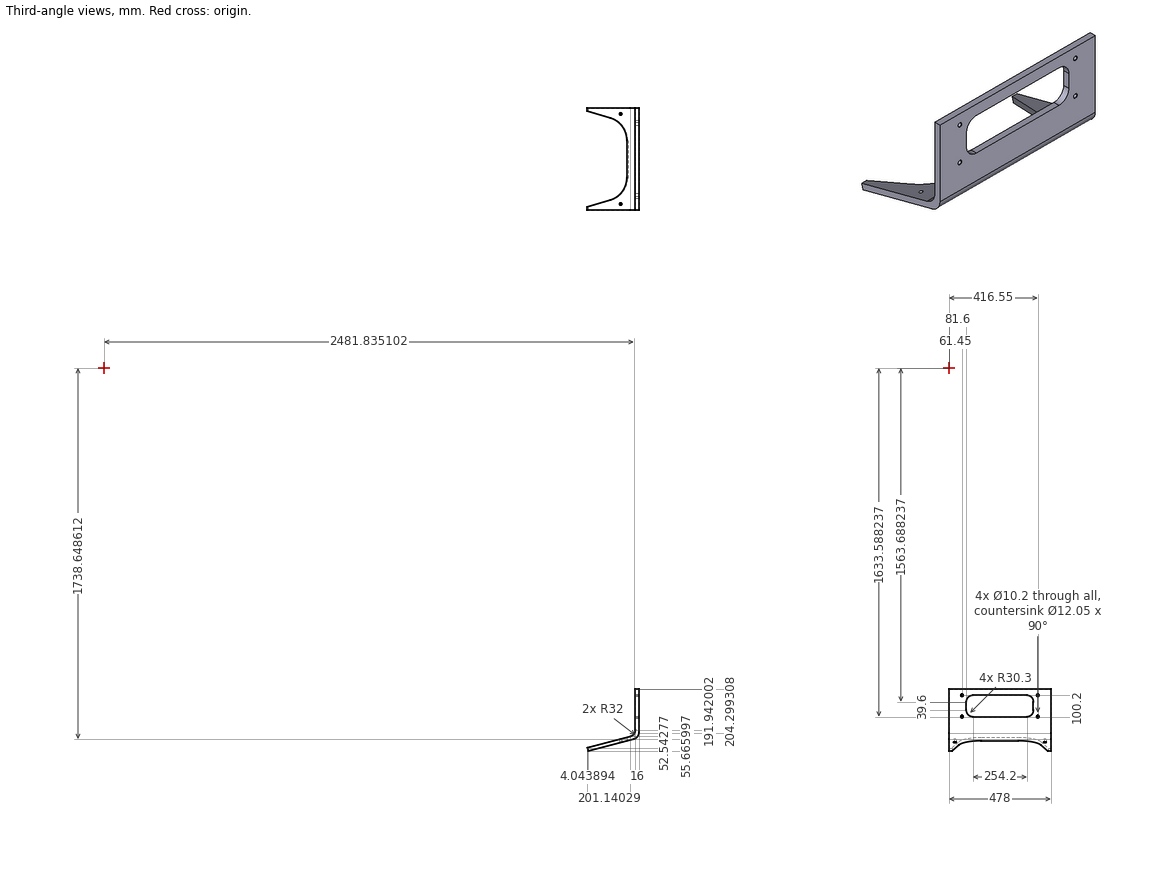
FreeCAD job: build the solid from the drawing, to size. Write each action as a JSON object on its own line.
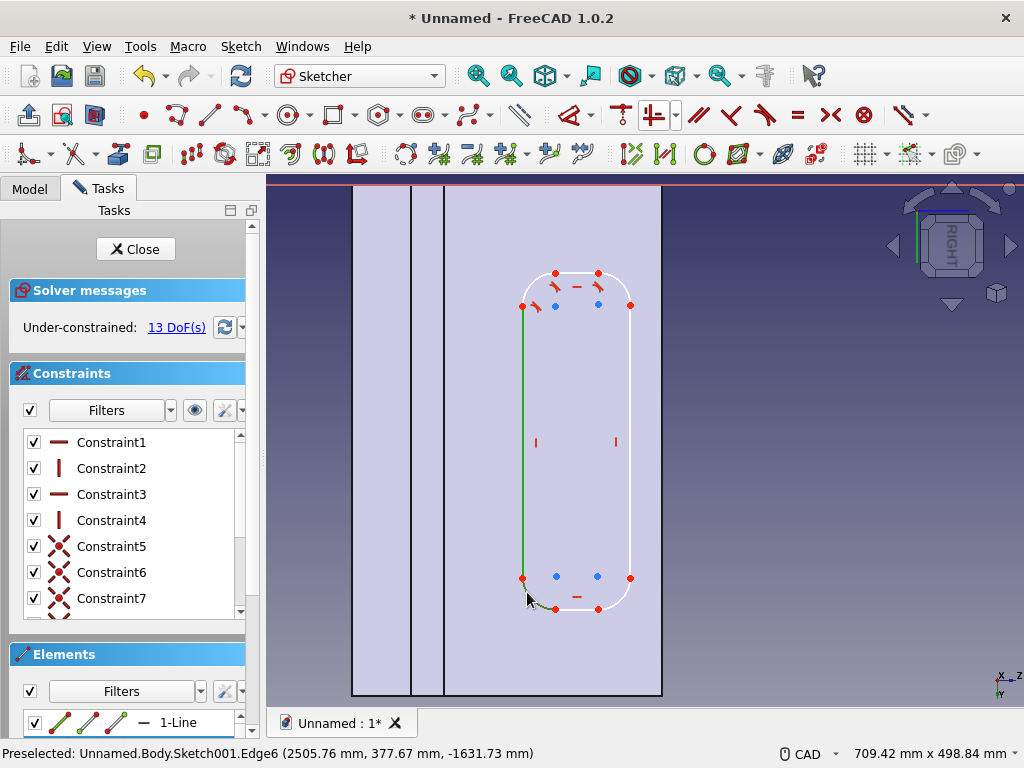
{"action": "left_click", "coordinate": [765, 116]}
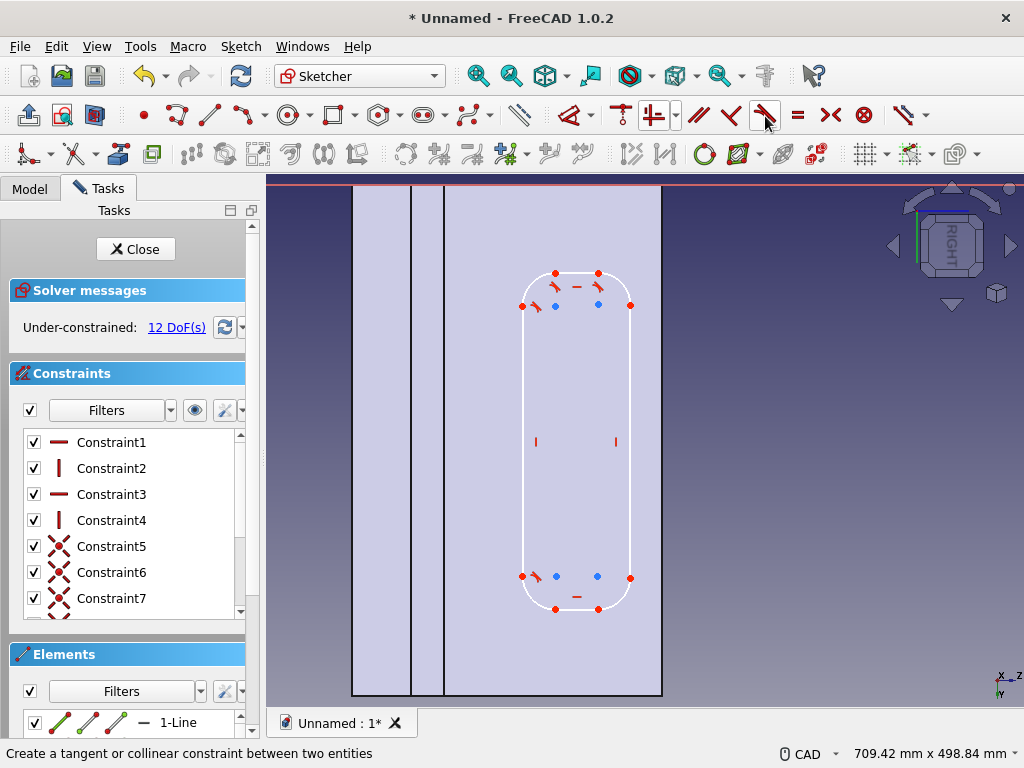
{"action": "left_click", "coordinate": [569, 610]}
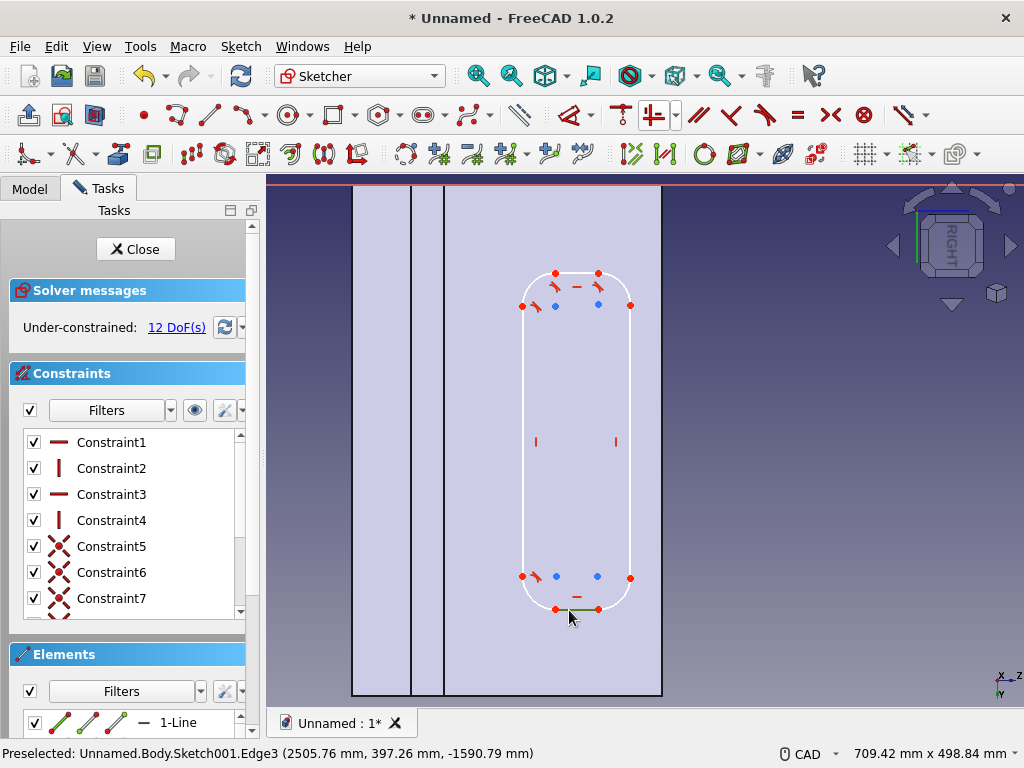
{"action": "left_click", "coordinate": [526, 591]}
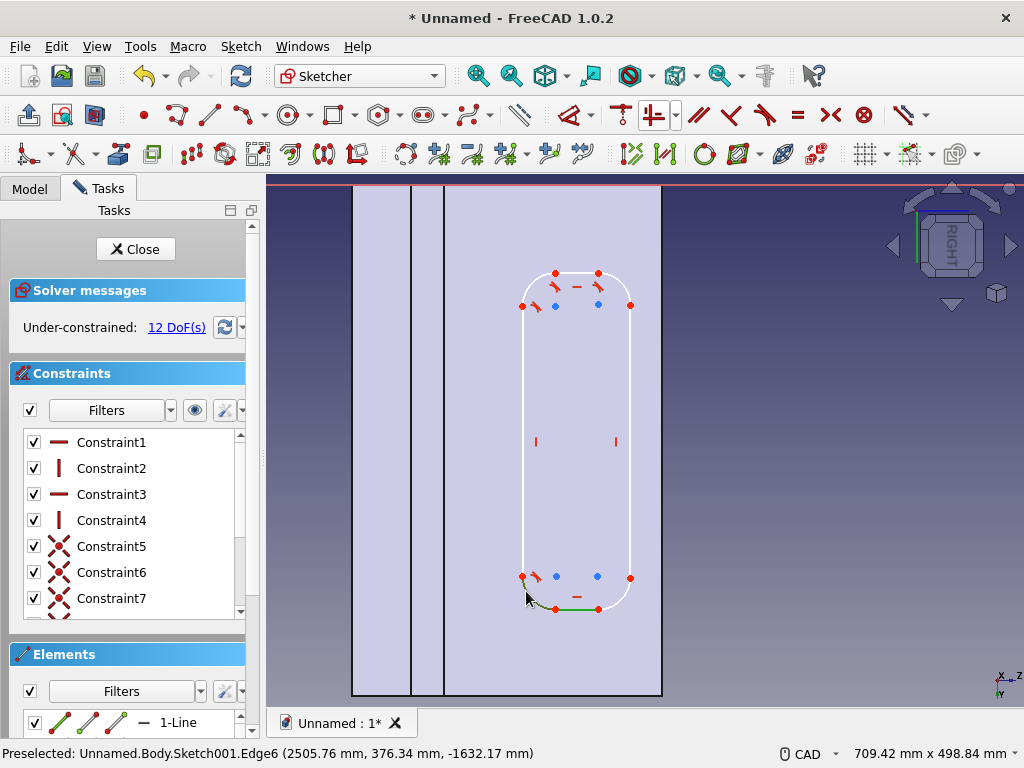
{"action": "left_click", "coordinate": [765, 116]}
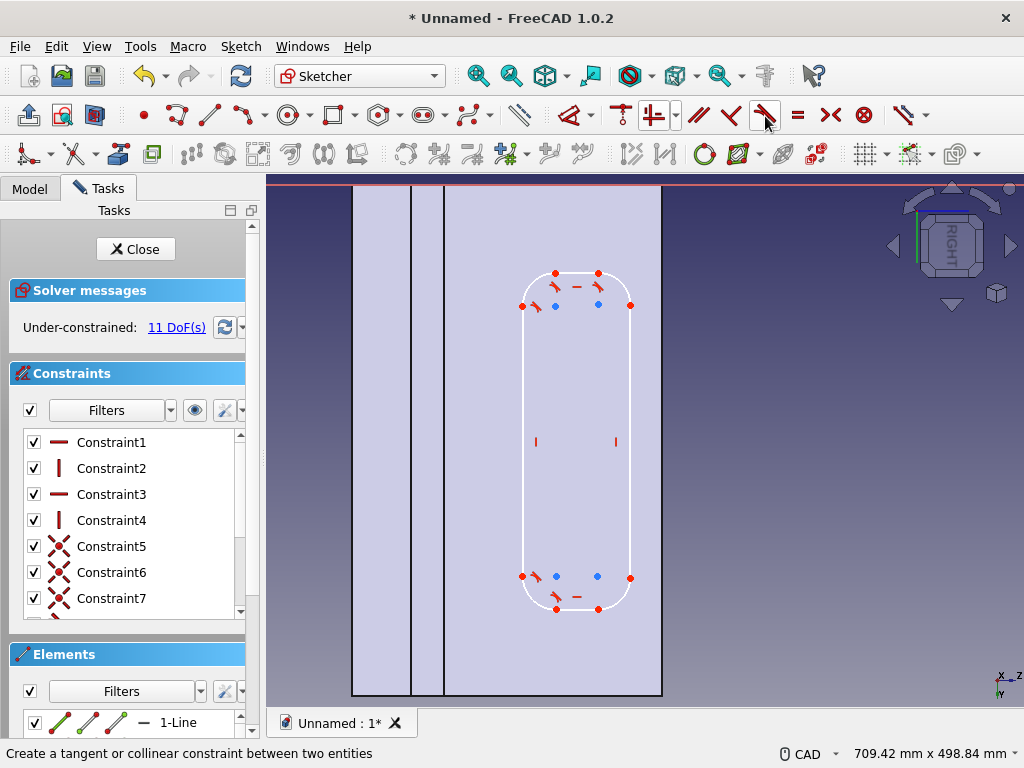
{"action": "left_click", "coordinate": [569, 610]}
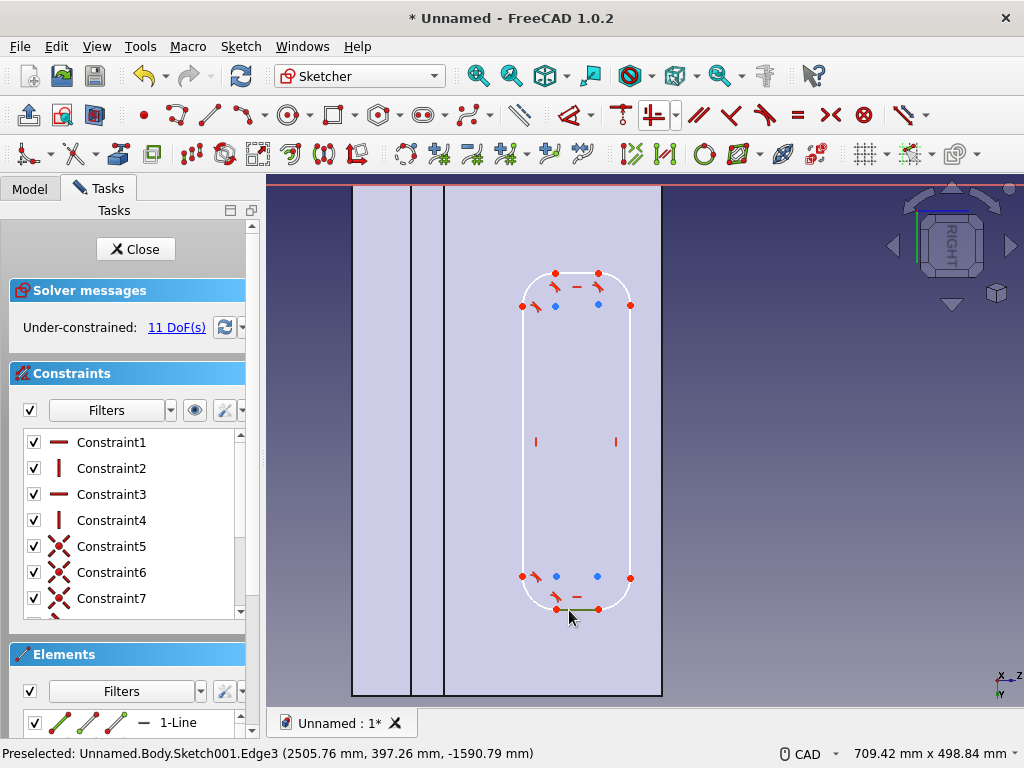
{"action": "left_click", "coordinate": [613, 606]}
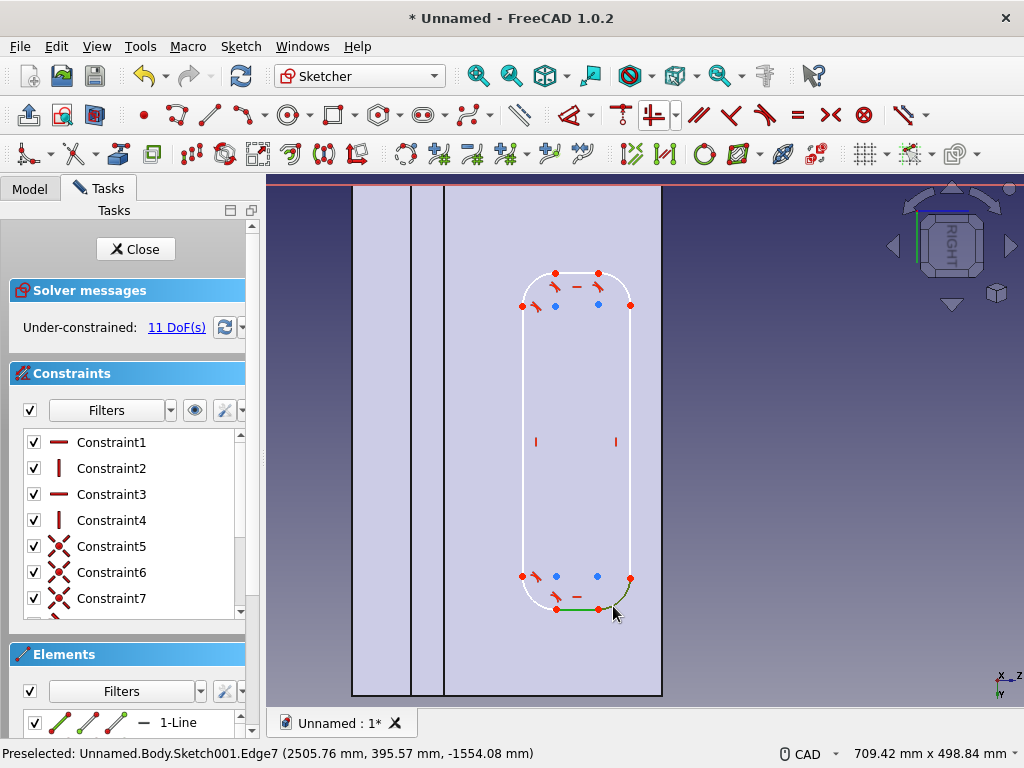
{"action": "left_click", "coordinate": [765, 116]}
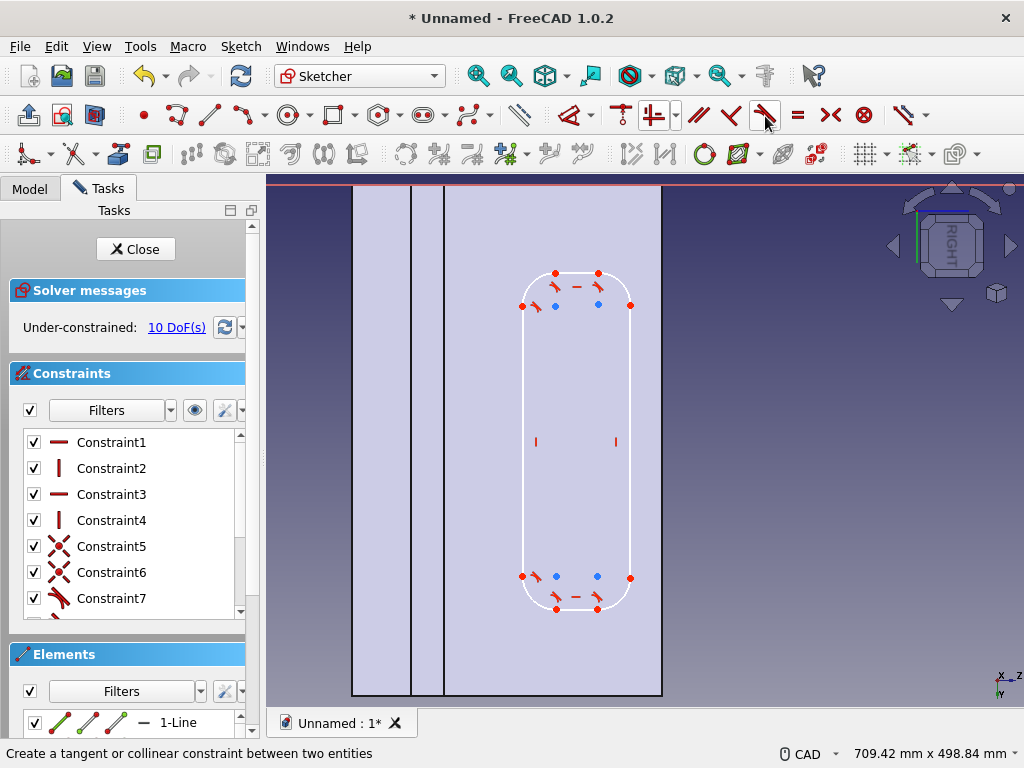
{"action": "left_click", "coordinate": [630, 496]}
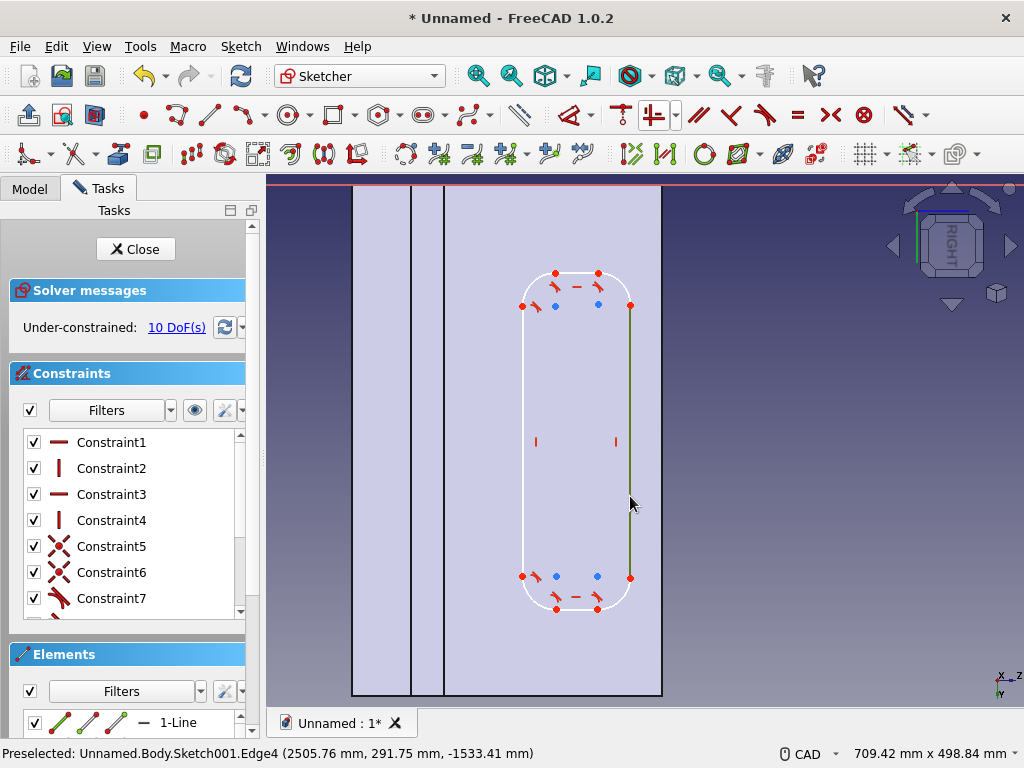
{"action": "left_click", "coordinate": [612, 606]}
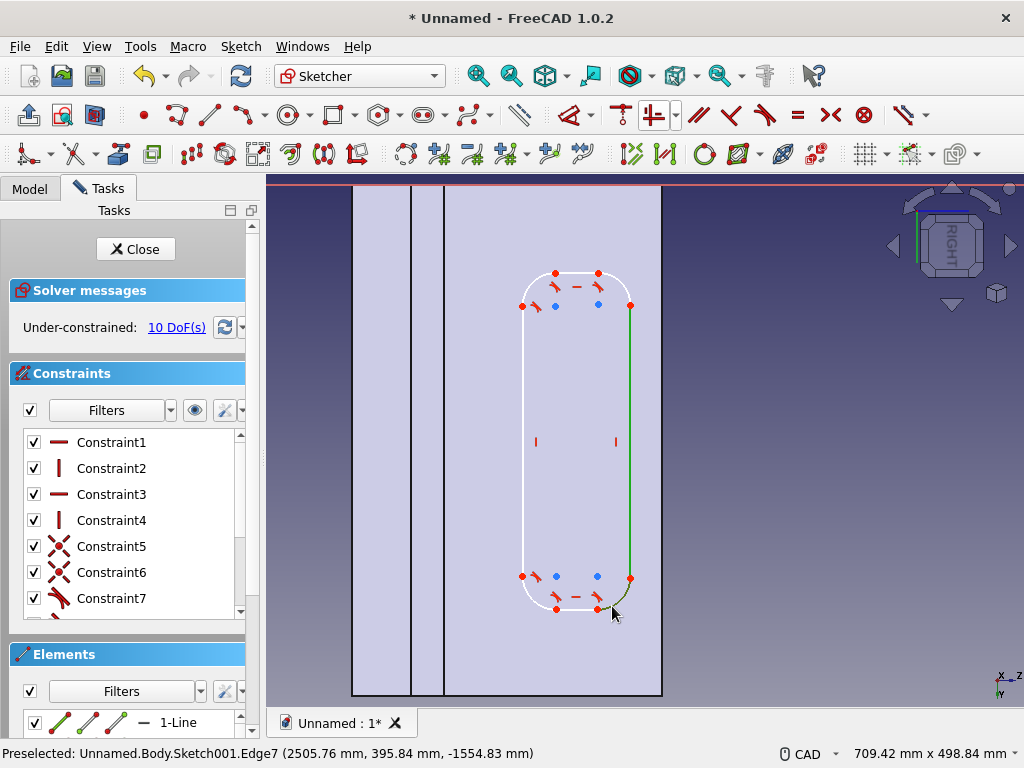
{"action": "left_click", "coordinate": [765, 116]}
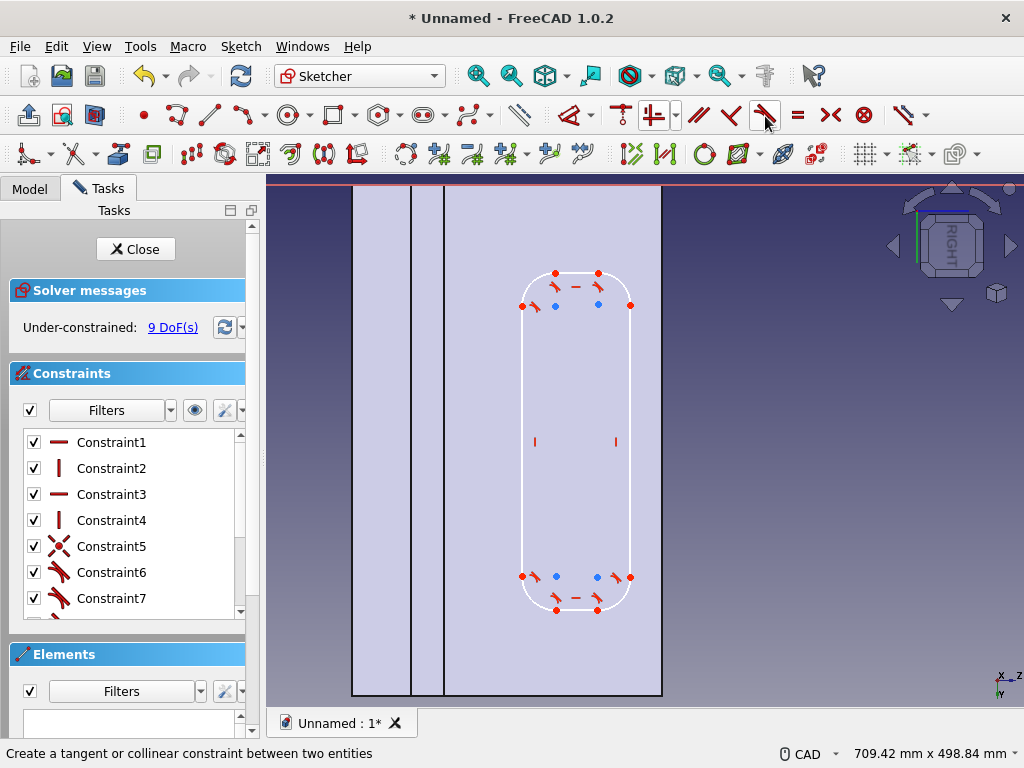
{"action": "left_click", "coordinate": [630, 496]}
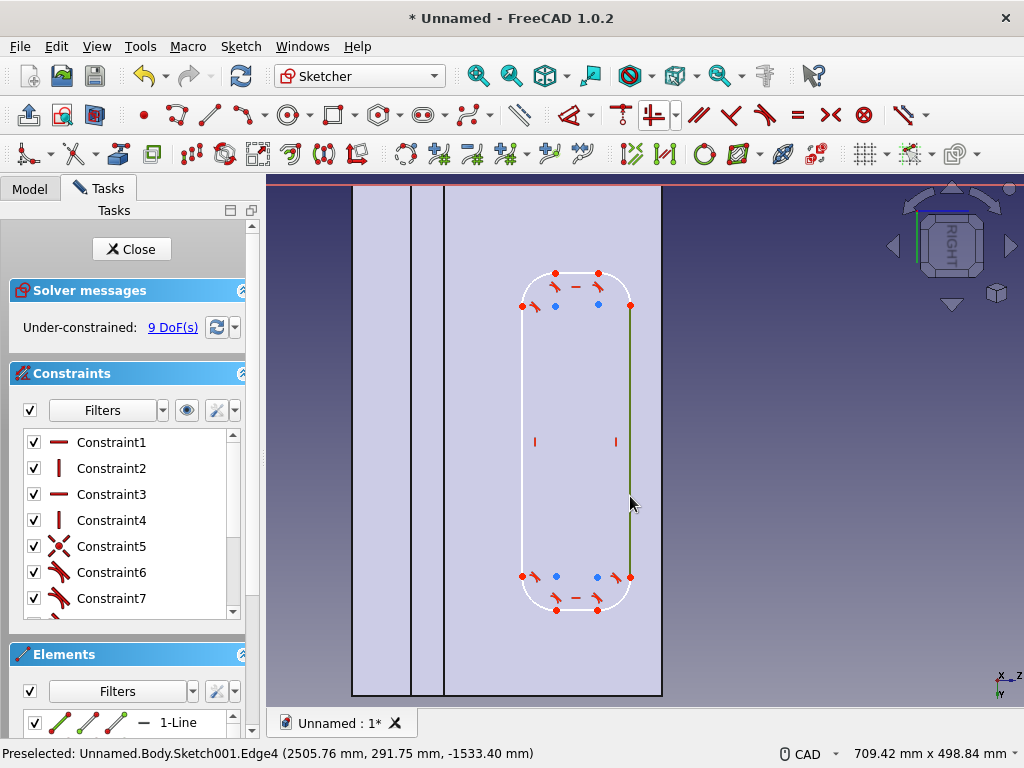
{"action": "left_click", "coordinate": [627, 291]}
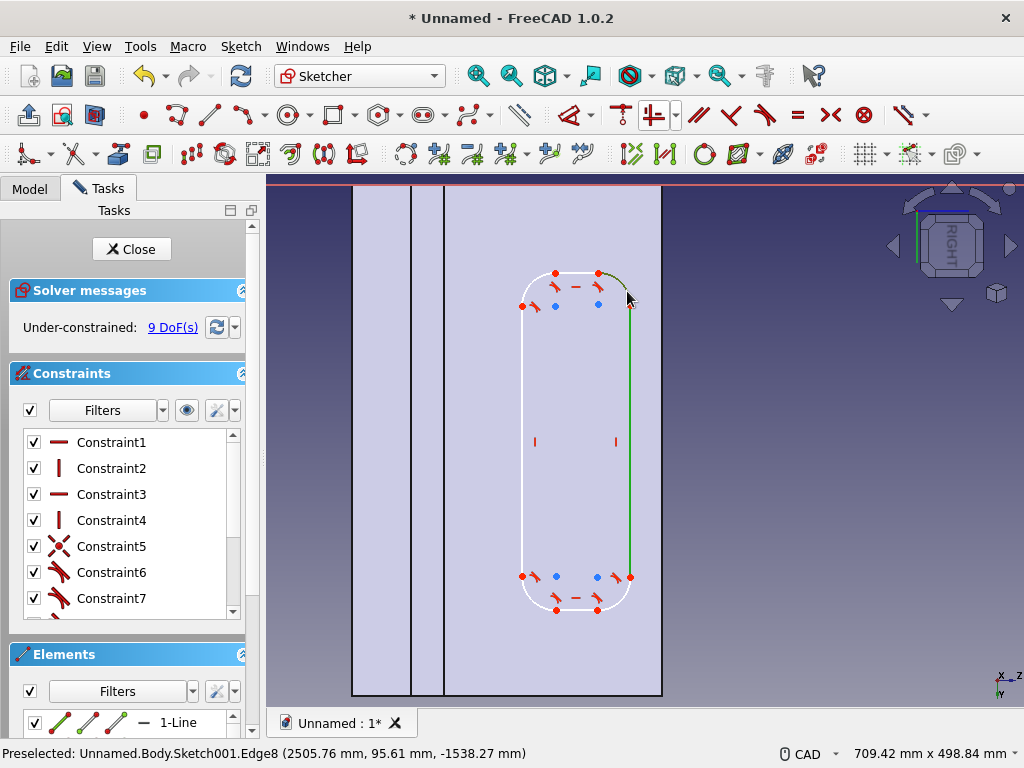
{"action": "left_click", "coordinate": [765, 116]}